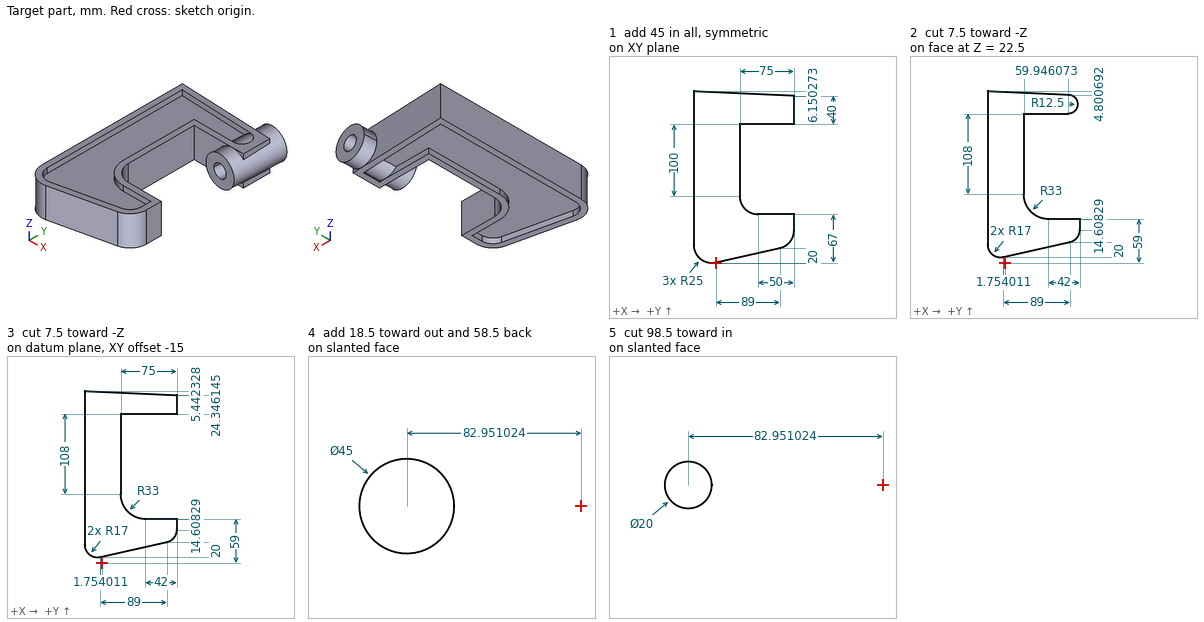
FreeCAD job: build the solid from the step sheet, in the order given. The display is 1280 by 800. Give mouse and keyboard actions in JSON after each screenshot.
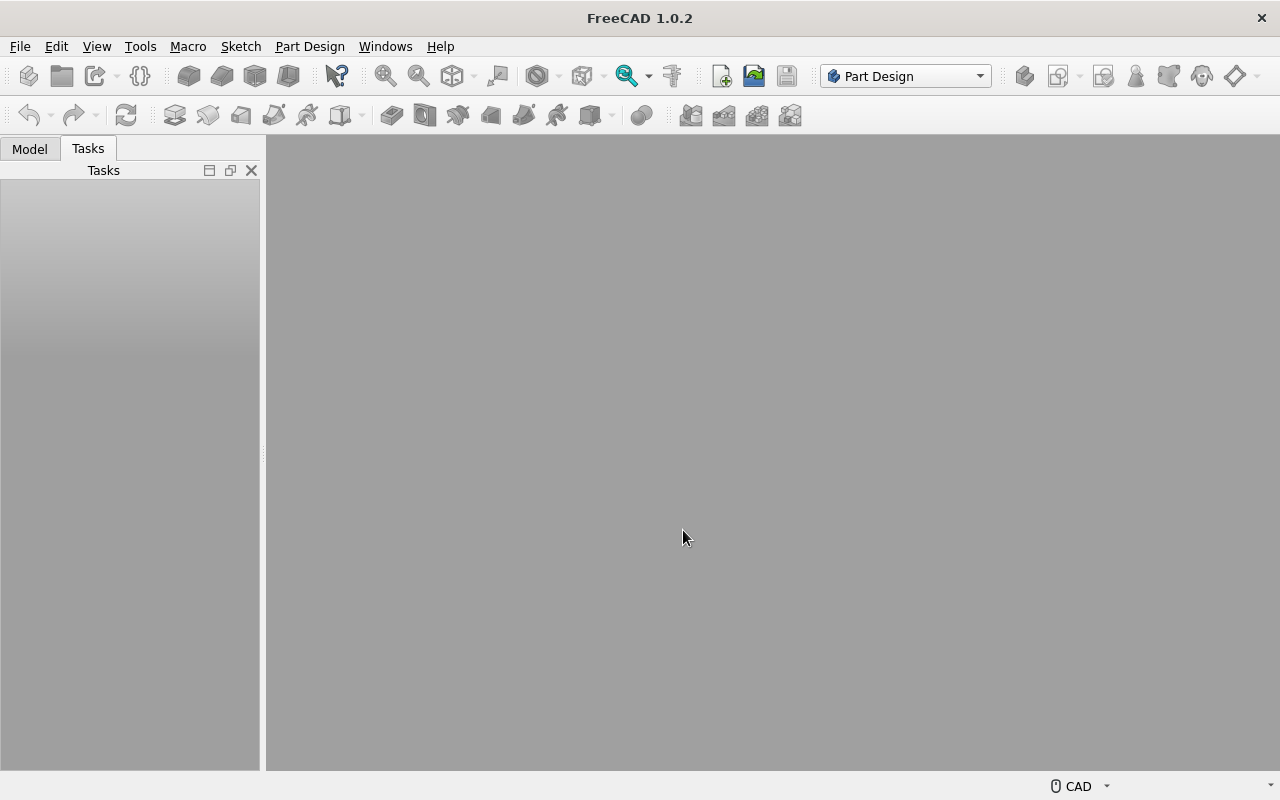
{"action": "left_click", "coordinate": [721, 76]}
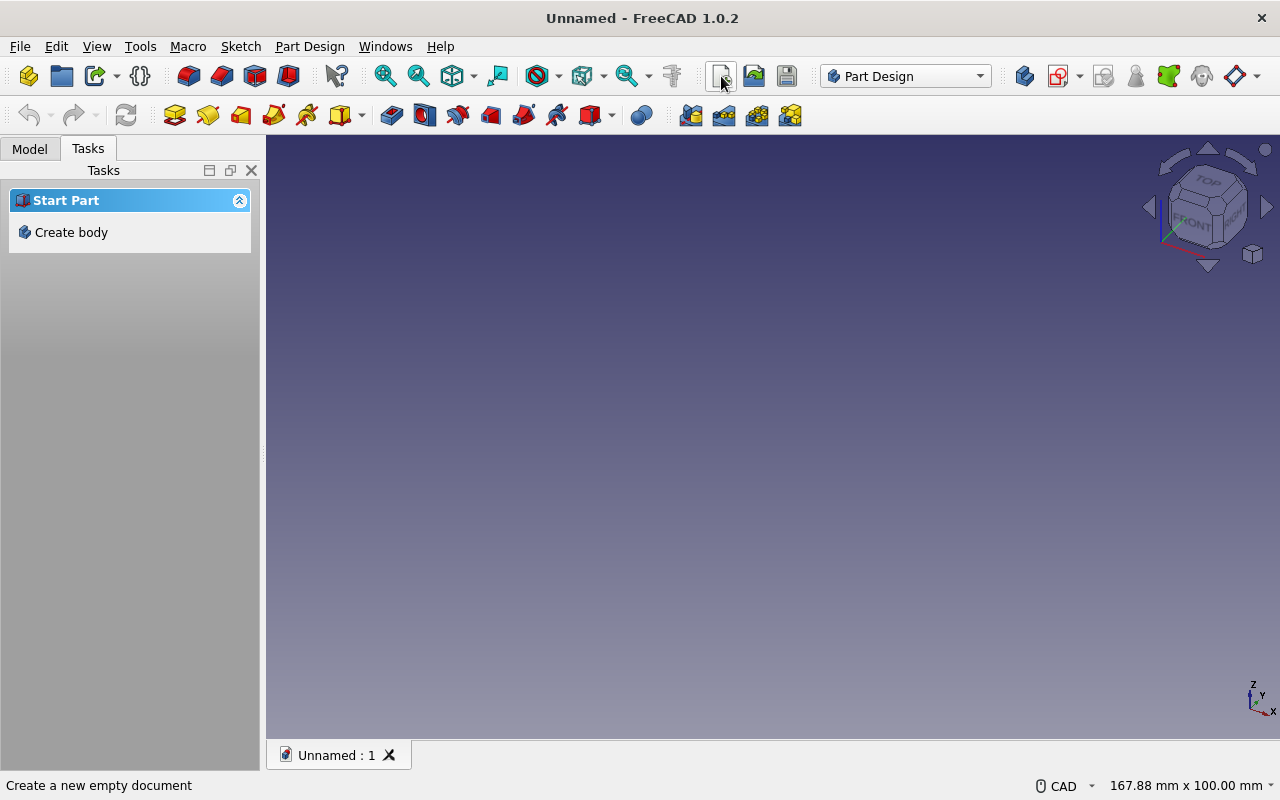
{"action": "left_click", "coordinate": [1058, 76]}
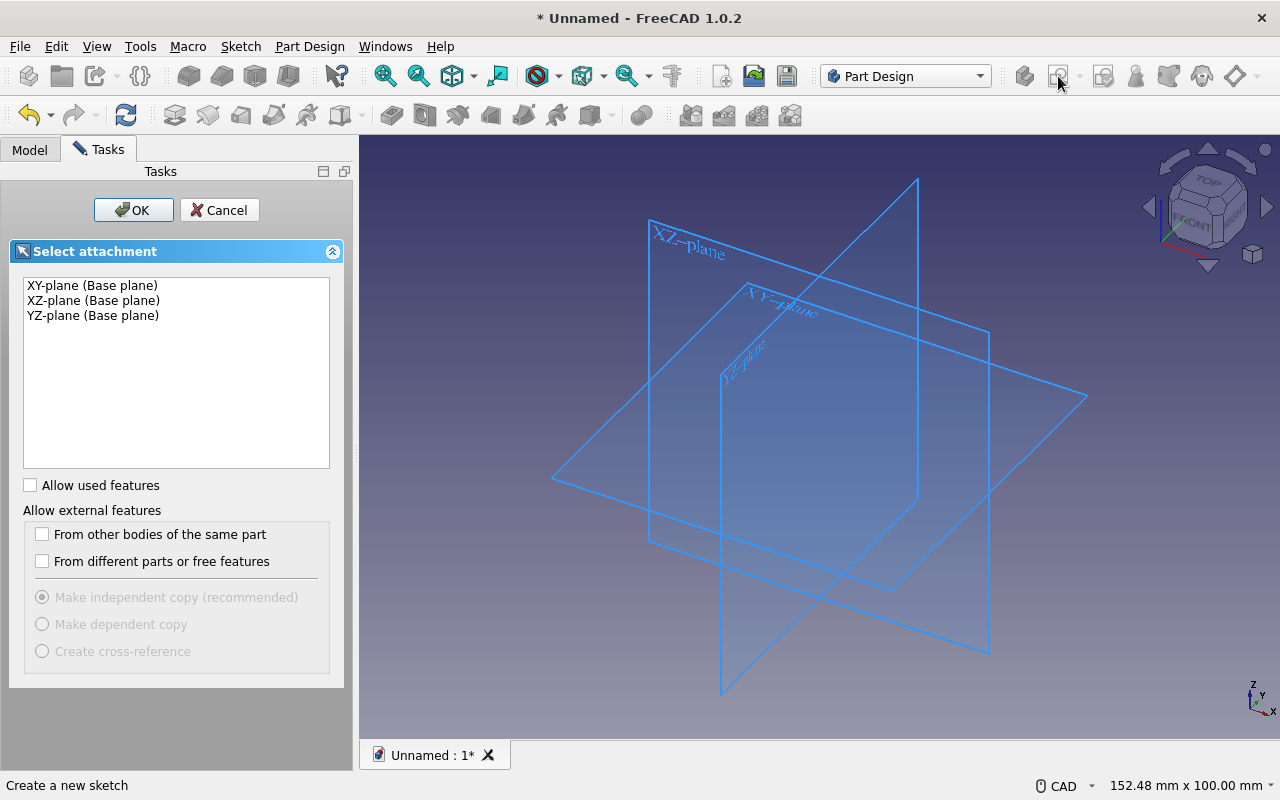
{"action": "left_click", "coordinate": [84, 286]}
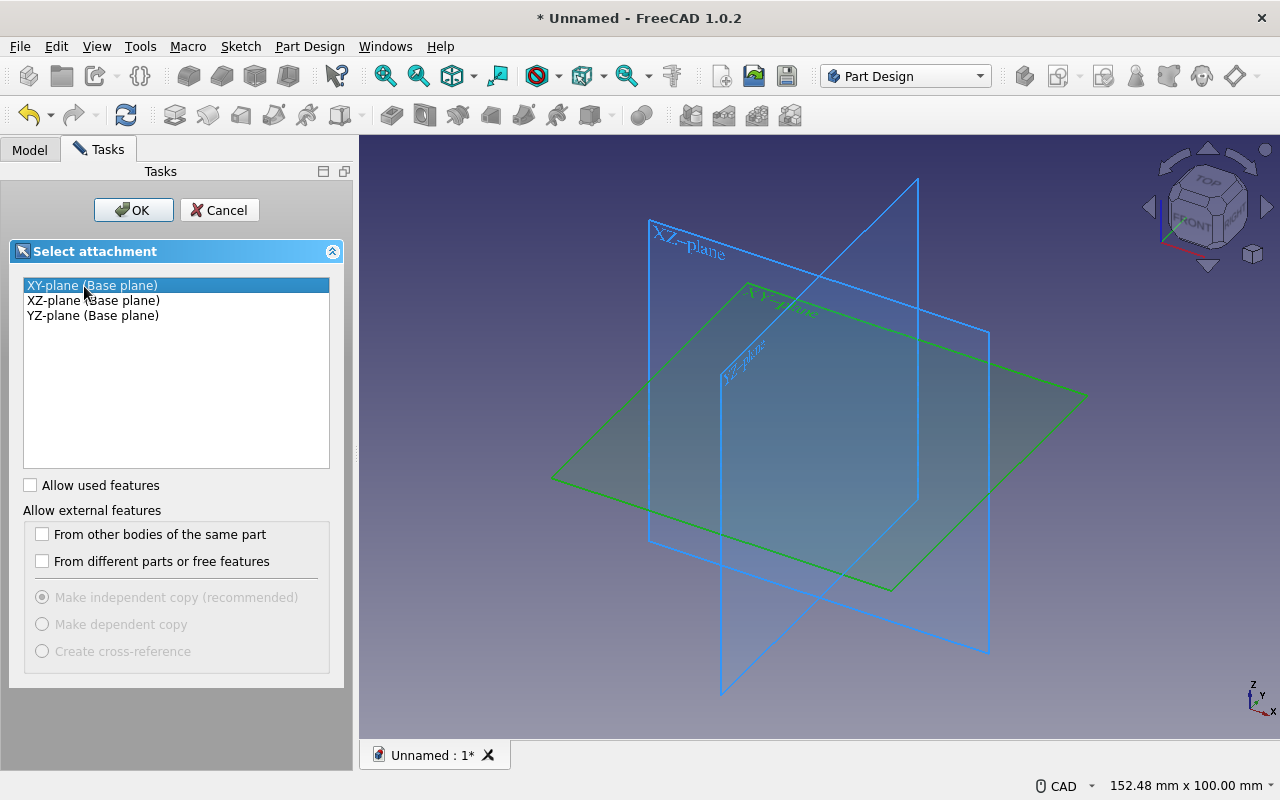
{"action": "left_click", "coordinate": [134, 210]}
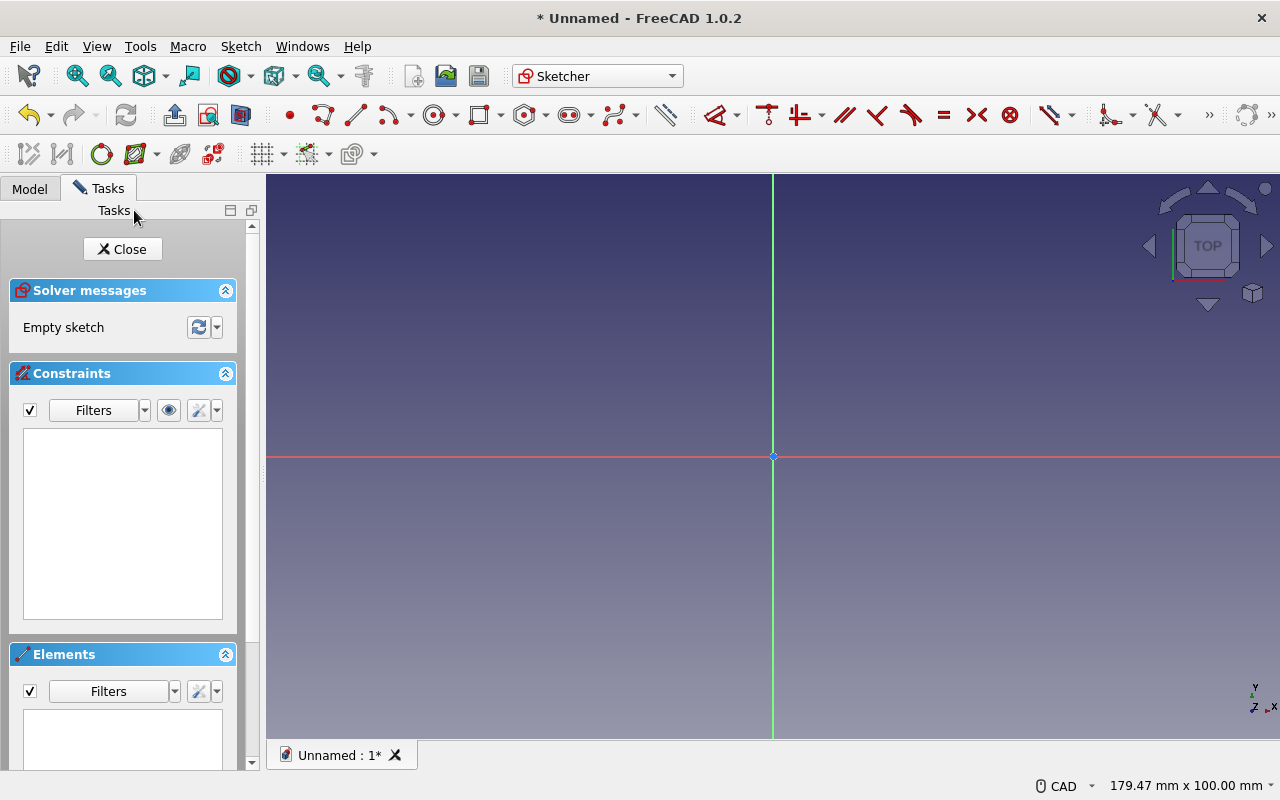
{"action": "scroll", "coordinate": [610, 677], "scroll_direction": "down", "scroll_amount": 7}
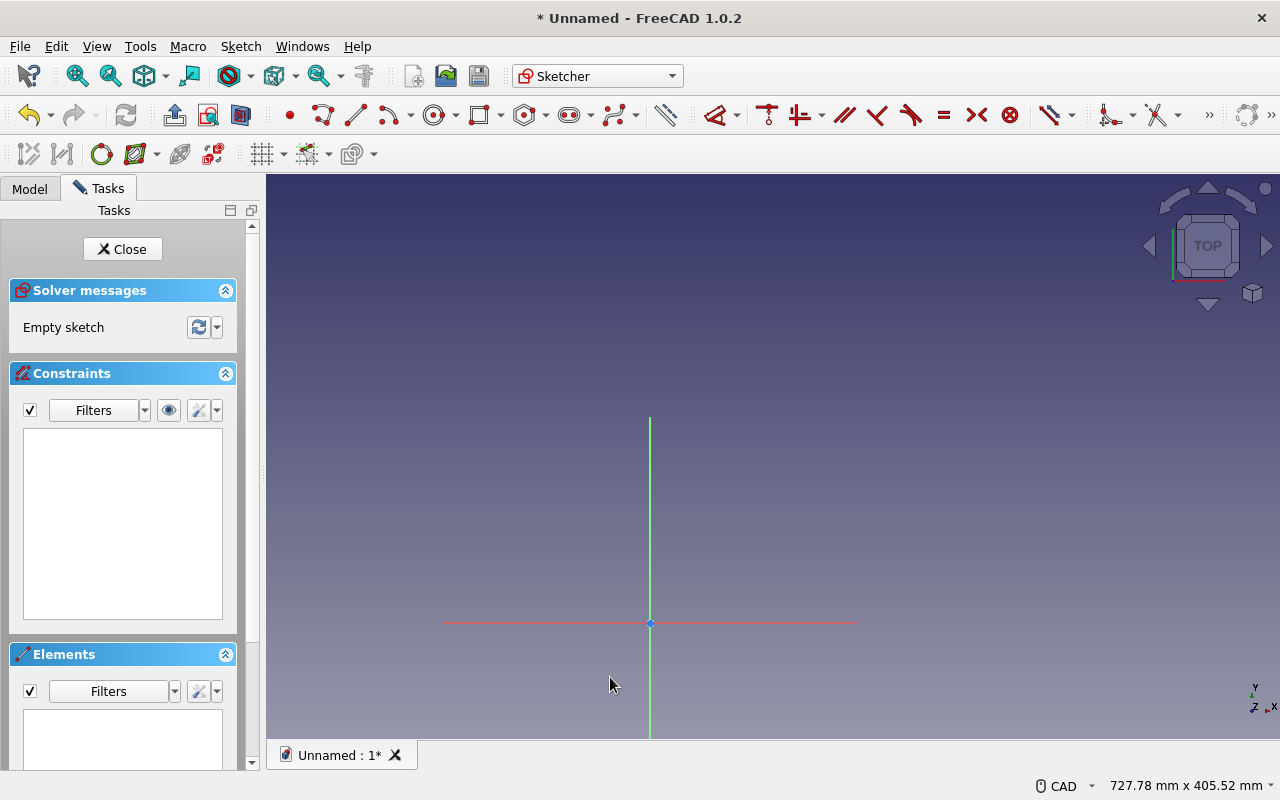
{"action": "left_click", "coordinate": [356, 116]}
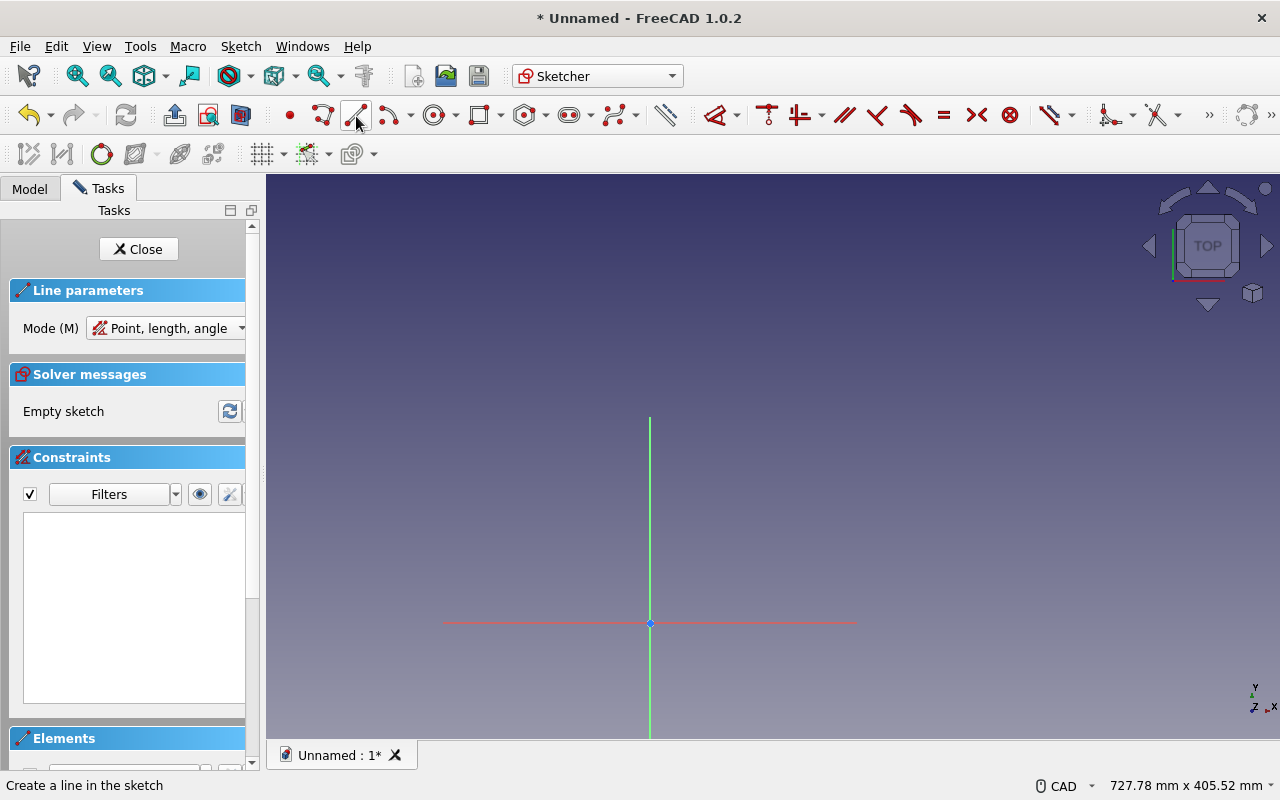
{"action": "left_click", "coordinate": [650, 623]}
{"action": "left_click", "coordinate": [774, 595]}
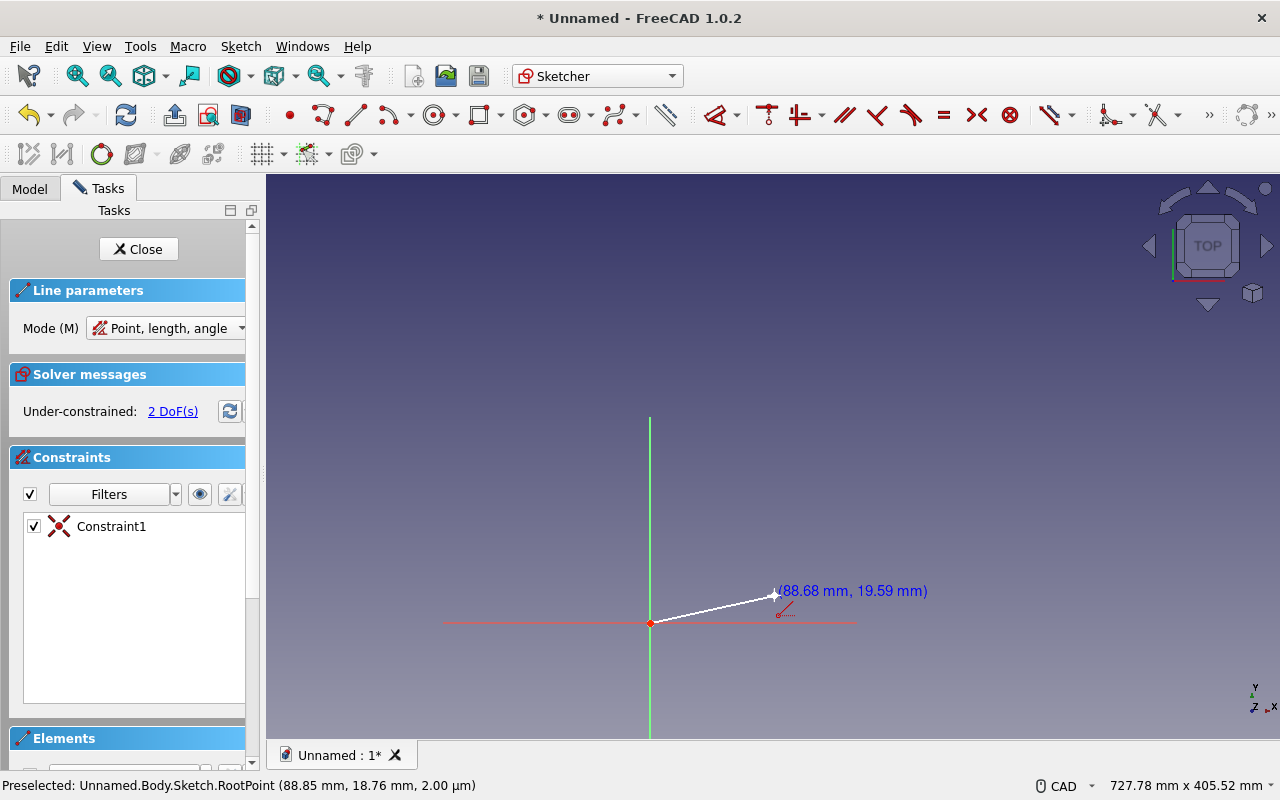
{"action": "key", "text": "g m"}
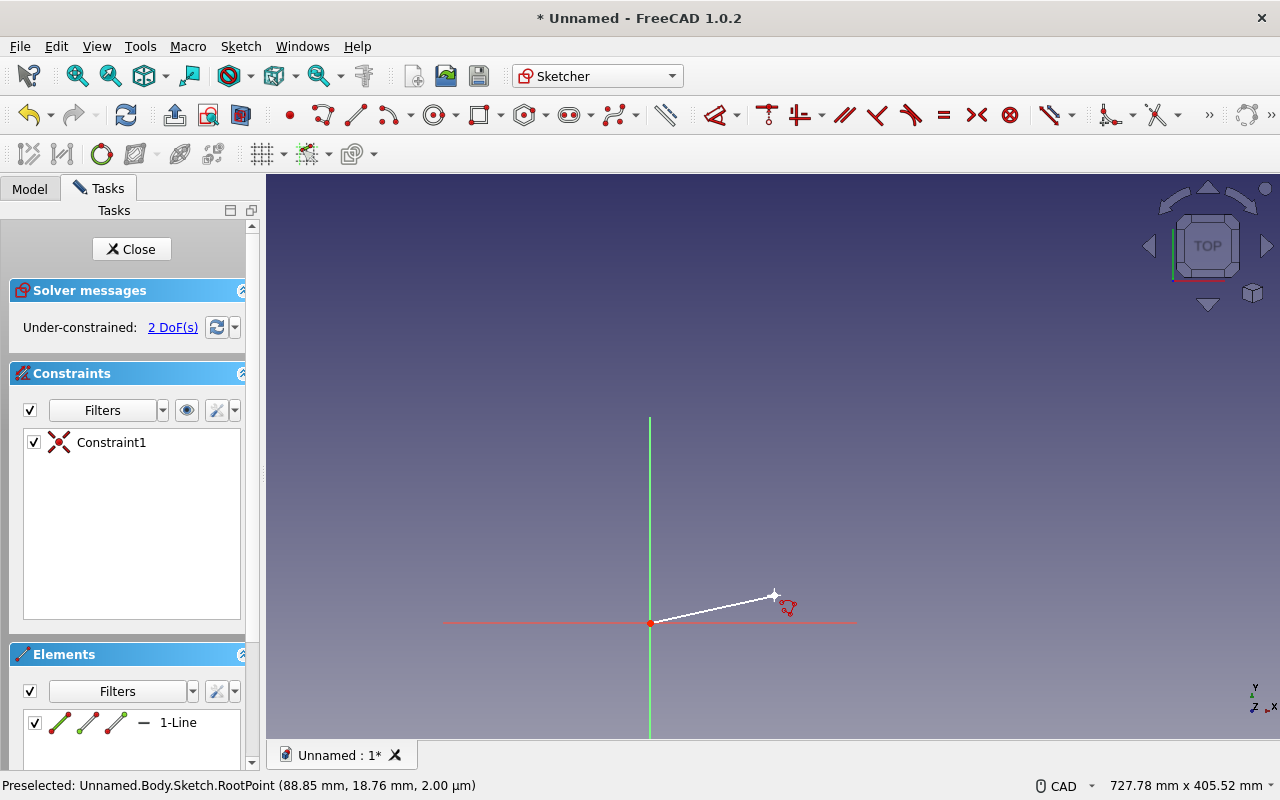
{"action": "left_click", "coordinate": [802, 561]}
{"action": "left_click", "coordinate": [802, 530]}
{"action": "left_click", "coordinate": [732, 530]}
{"action": "right_click", "coordinate": [732, 530]}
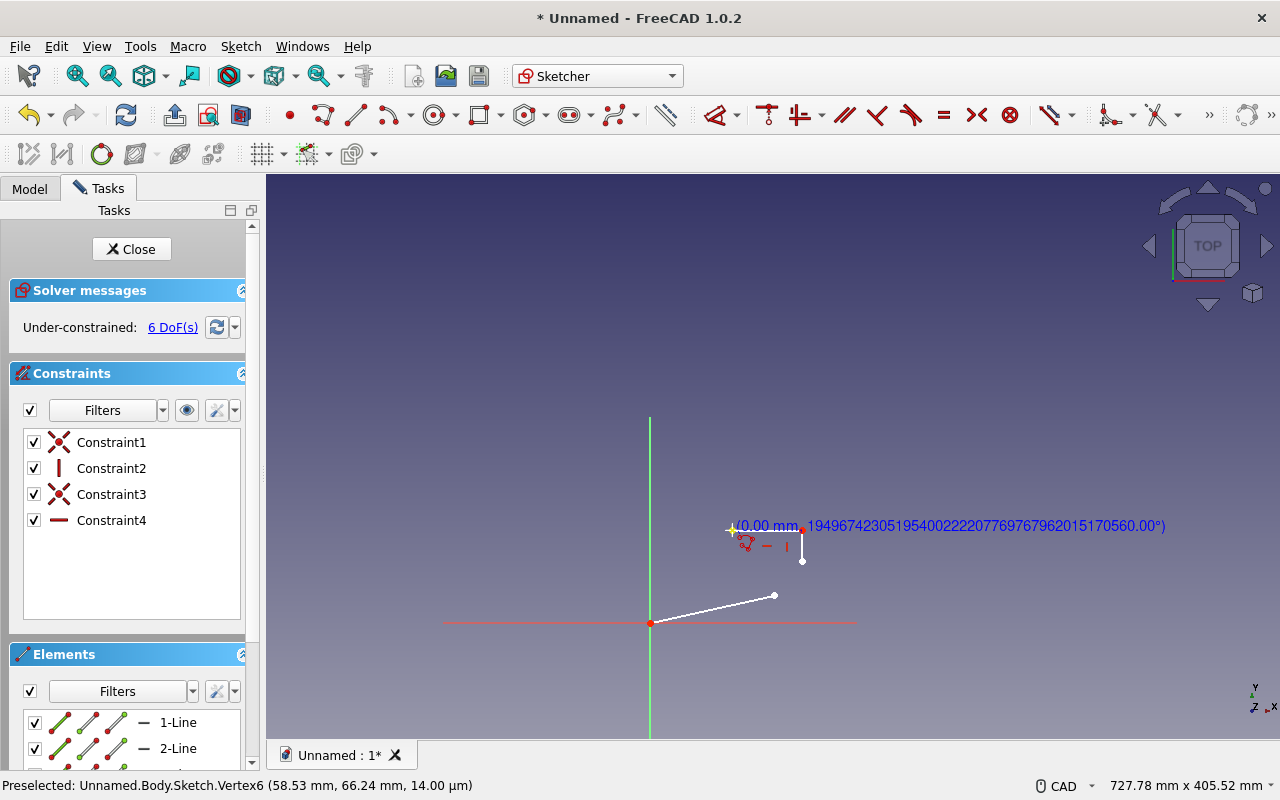
{"action": "left_click", "coordinate": [697, 495]}
{"action": "left_click", "coordinate": [697, 356]}
{"action": "left_click", "coordinate": [802, 356]}
{"action": "left_click", "coordinate": [802, 300]}
{"action": "left_click", "coordinate": [608, 290]}
{"action": "left_click", "coordinate": [608, 589]}
{"action": "right_click", "coordinate": [608, 589]}